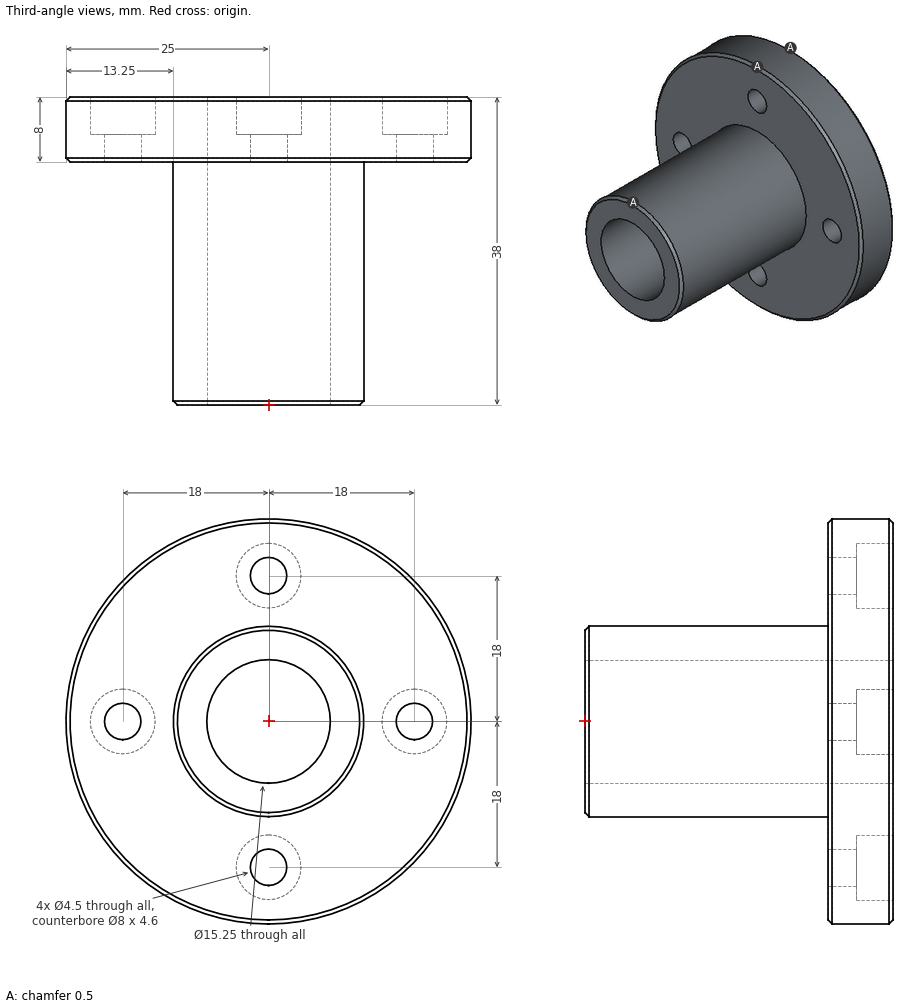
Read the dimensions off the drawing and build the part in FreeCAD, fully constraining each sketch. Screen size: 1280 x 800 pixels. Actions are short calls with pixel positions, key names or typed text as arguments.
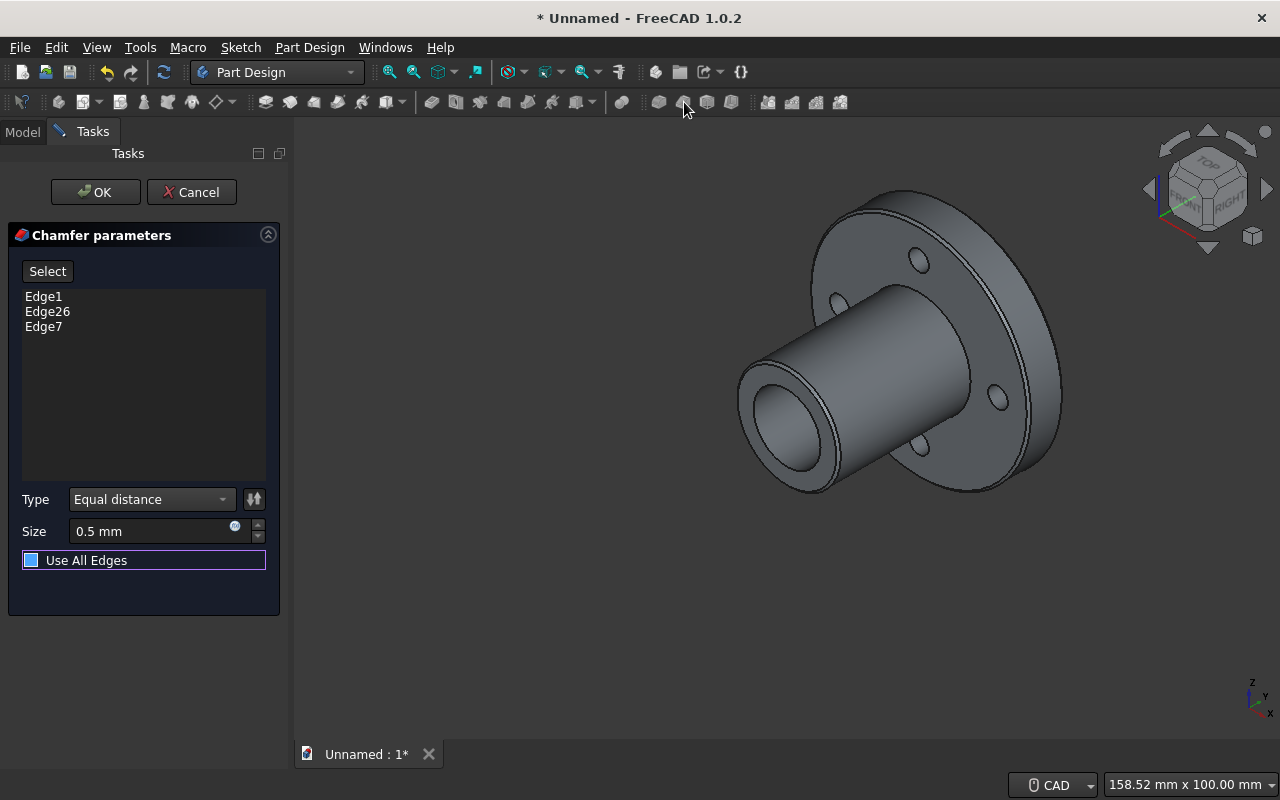
click(96, 192)